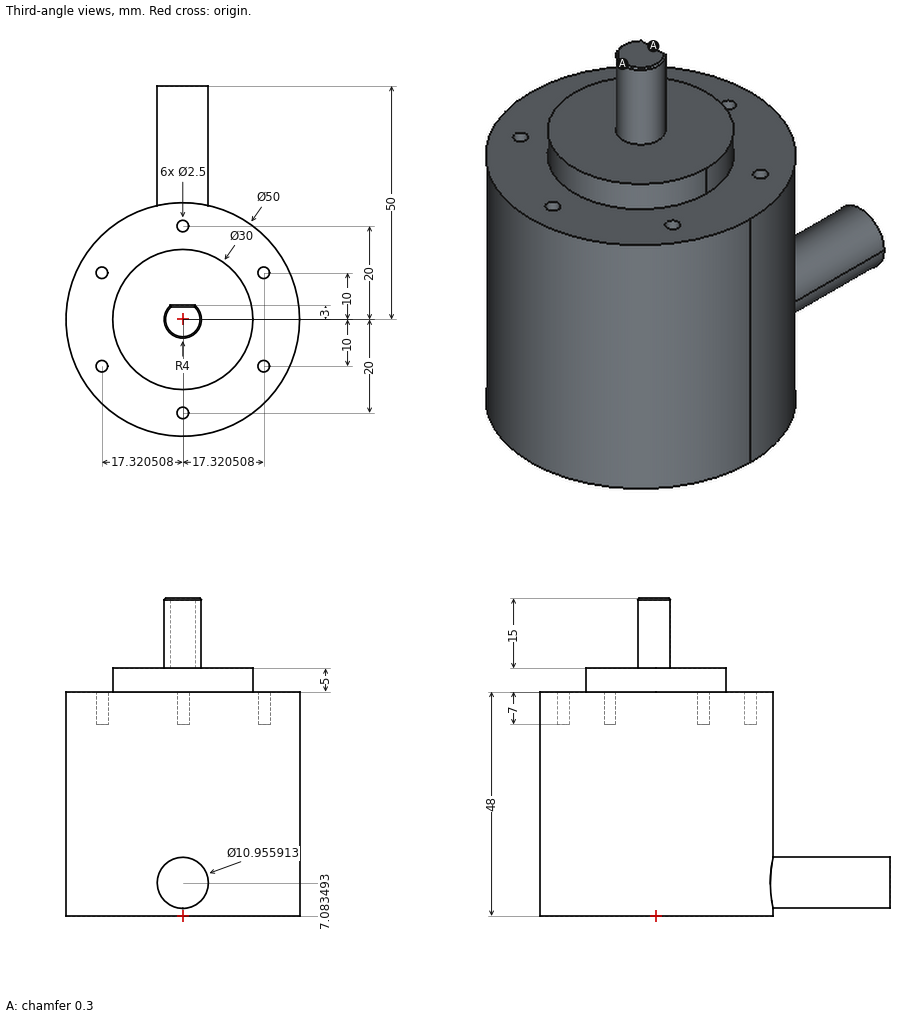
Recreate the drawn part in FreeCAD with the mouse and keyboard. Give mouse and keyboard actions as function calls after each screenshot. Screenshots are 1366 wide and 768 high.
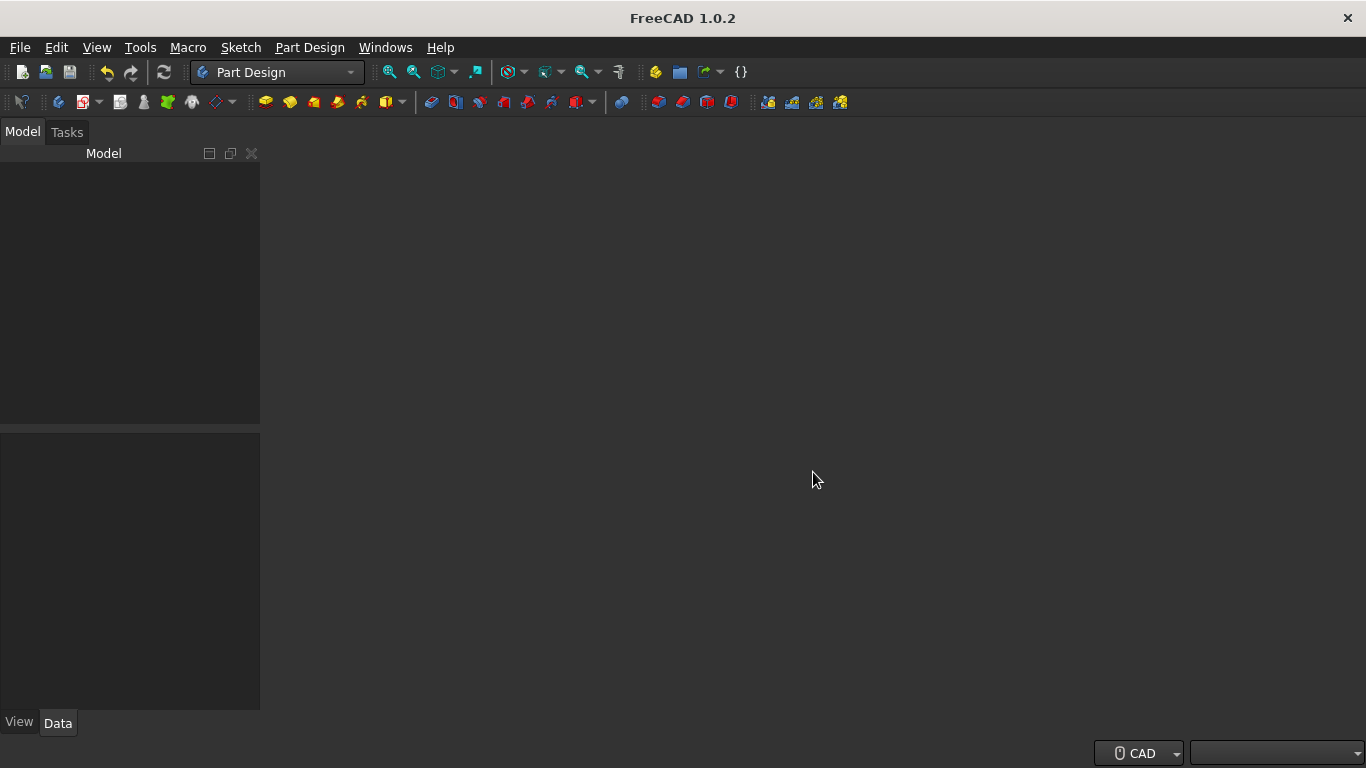
click(22, 72)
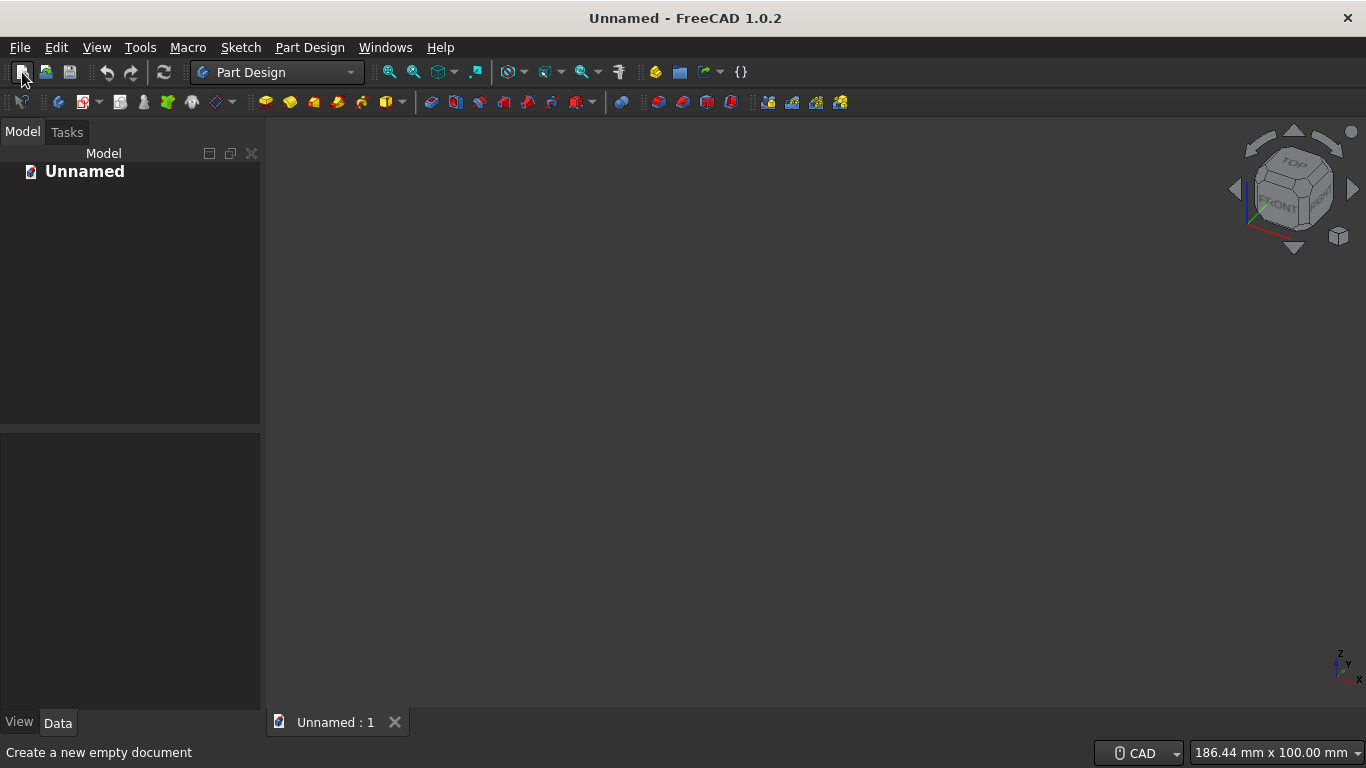
click(84, 102)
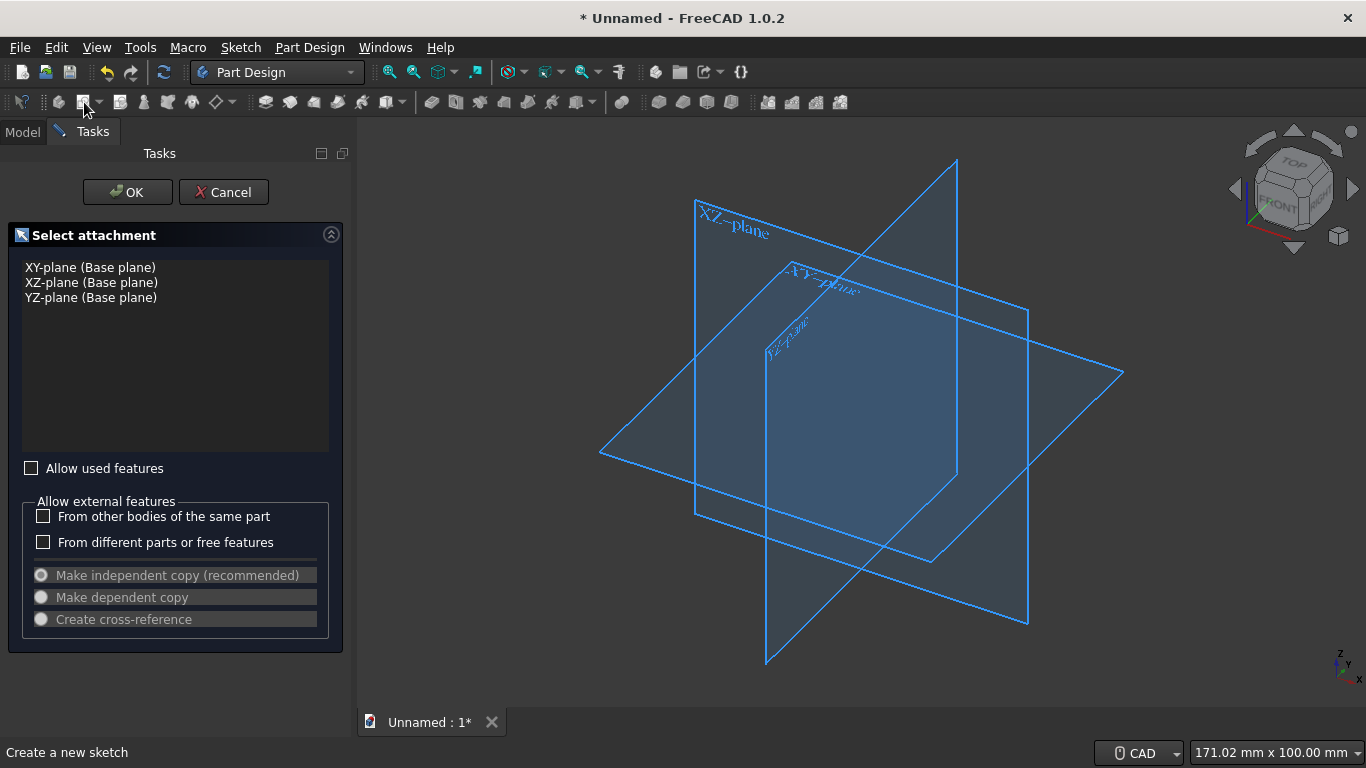
click(82, 268)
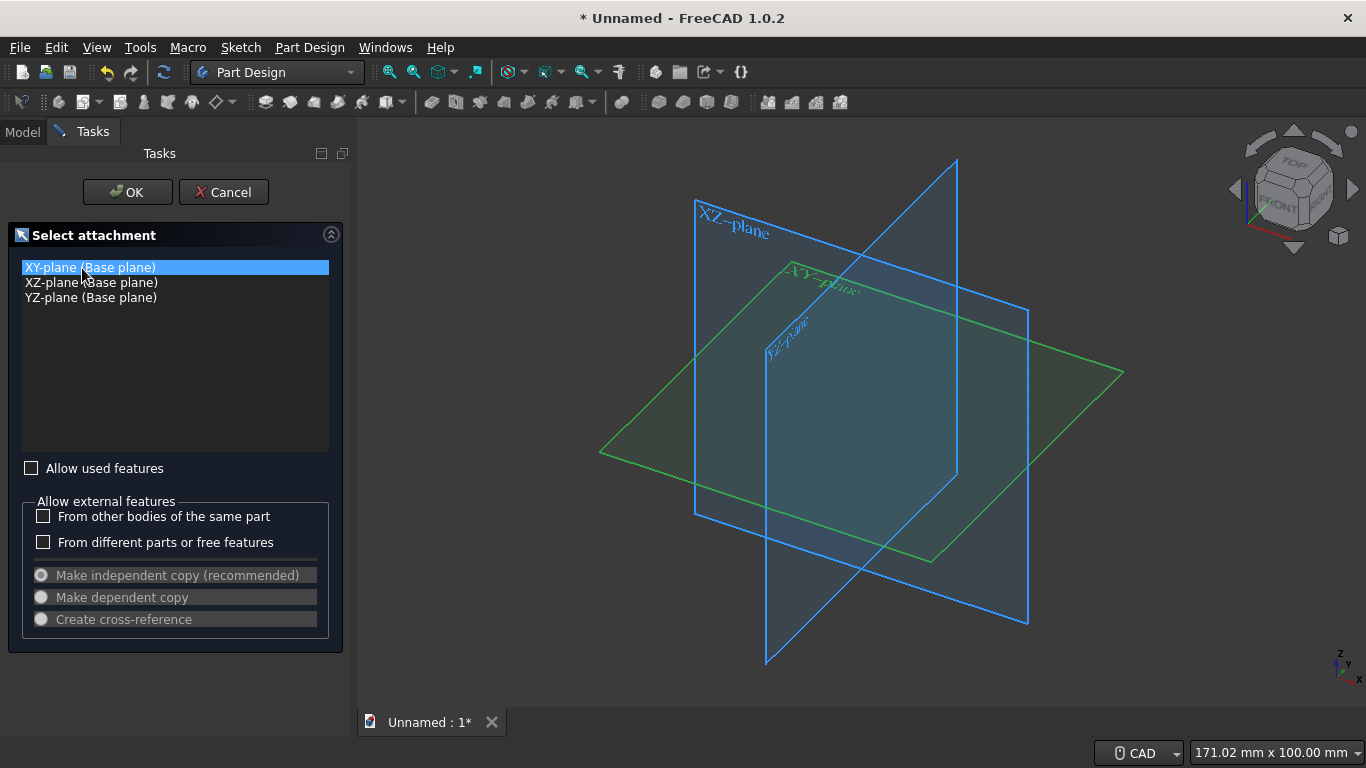
click(128, 192)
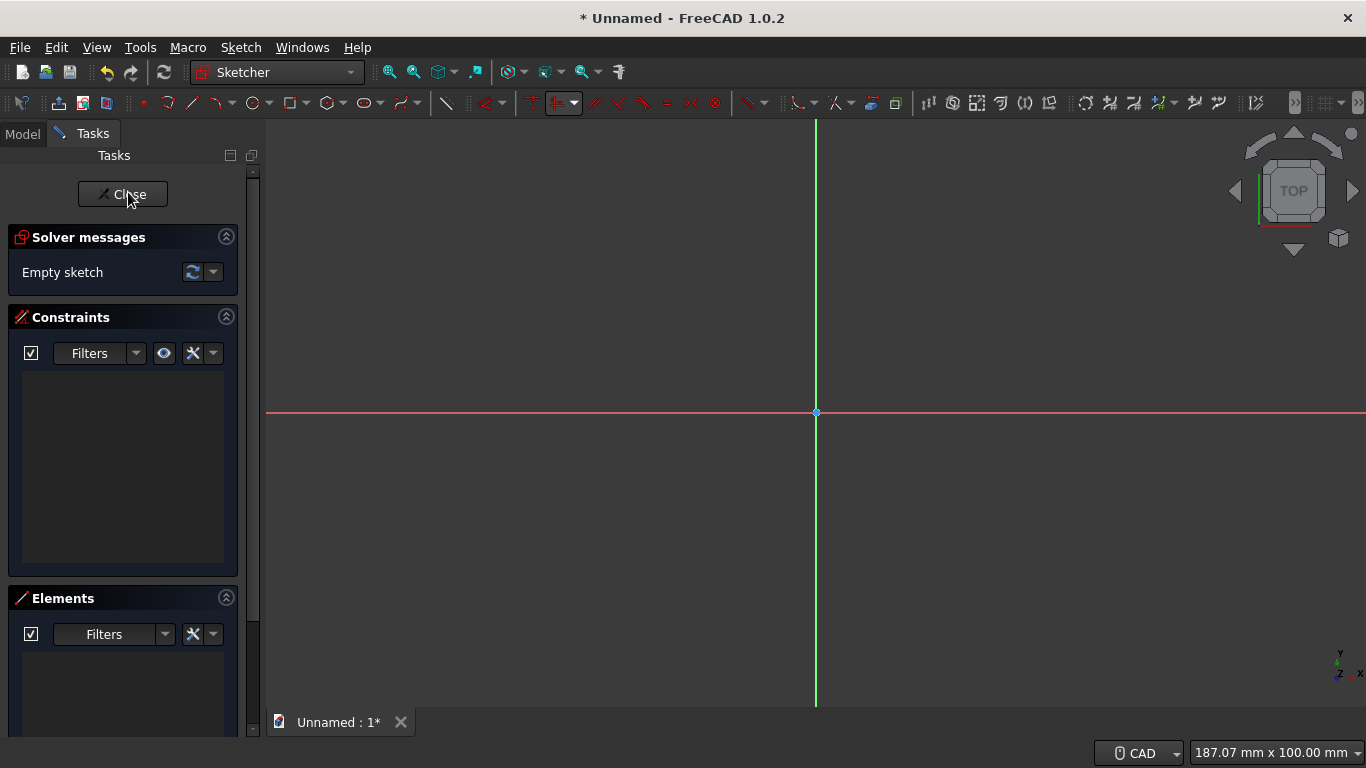
click(254, 104)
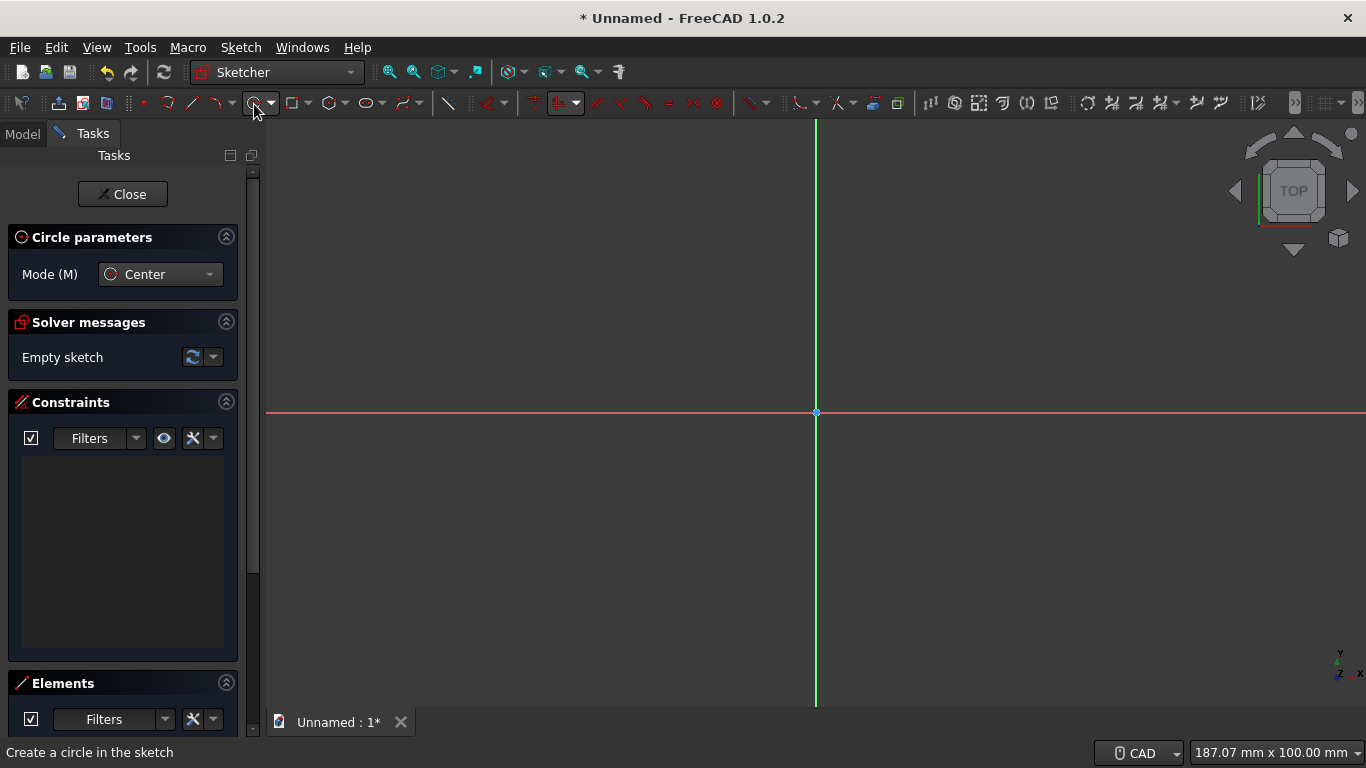
click(816, 413)
move(920, 309)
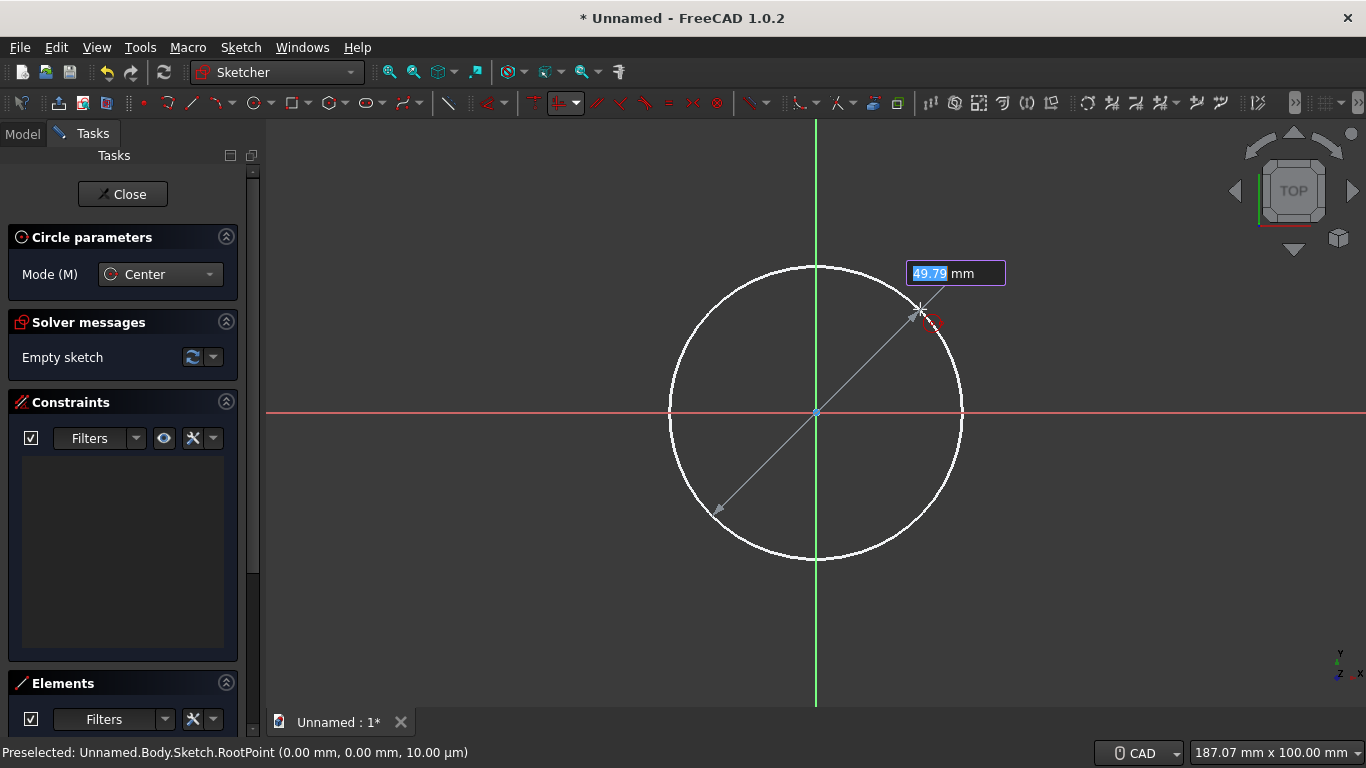
text(50)
key(Return)
key(Escape)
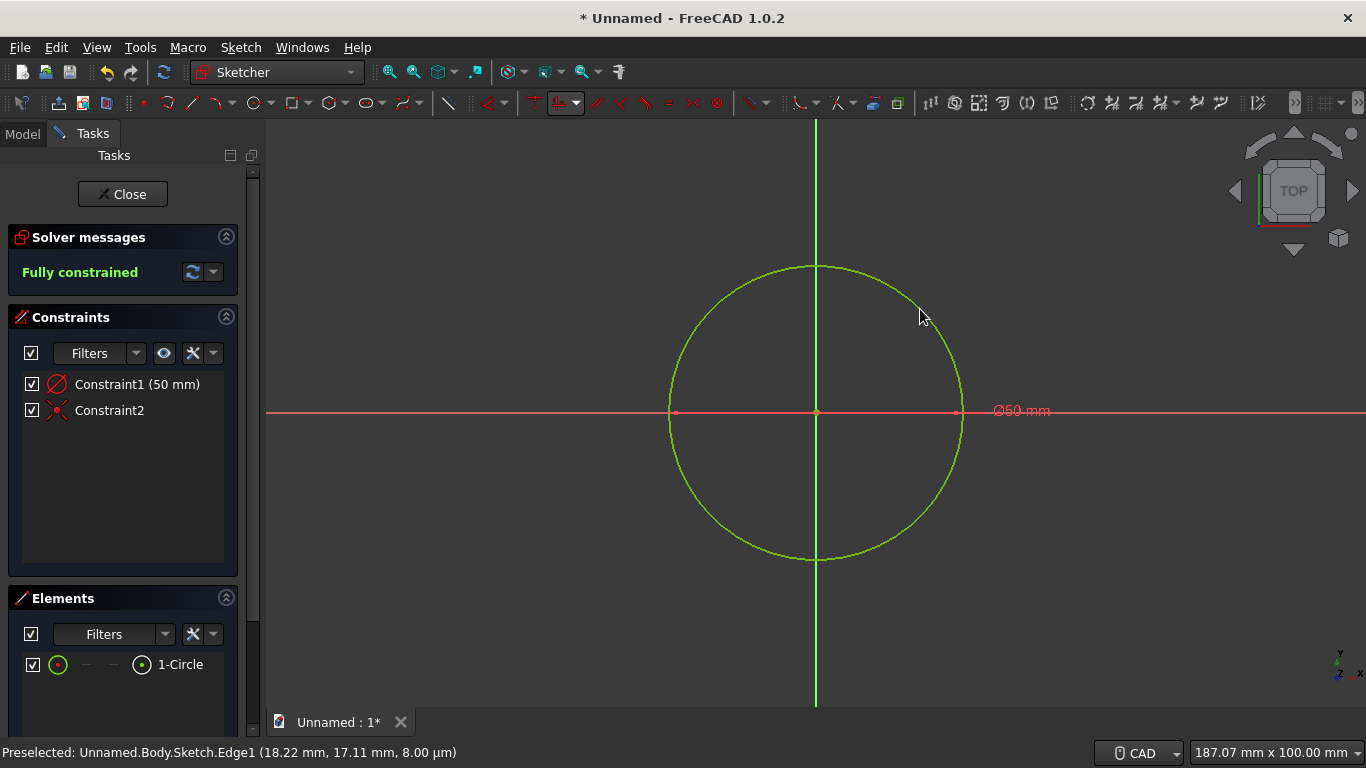
click(123, 194)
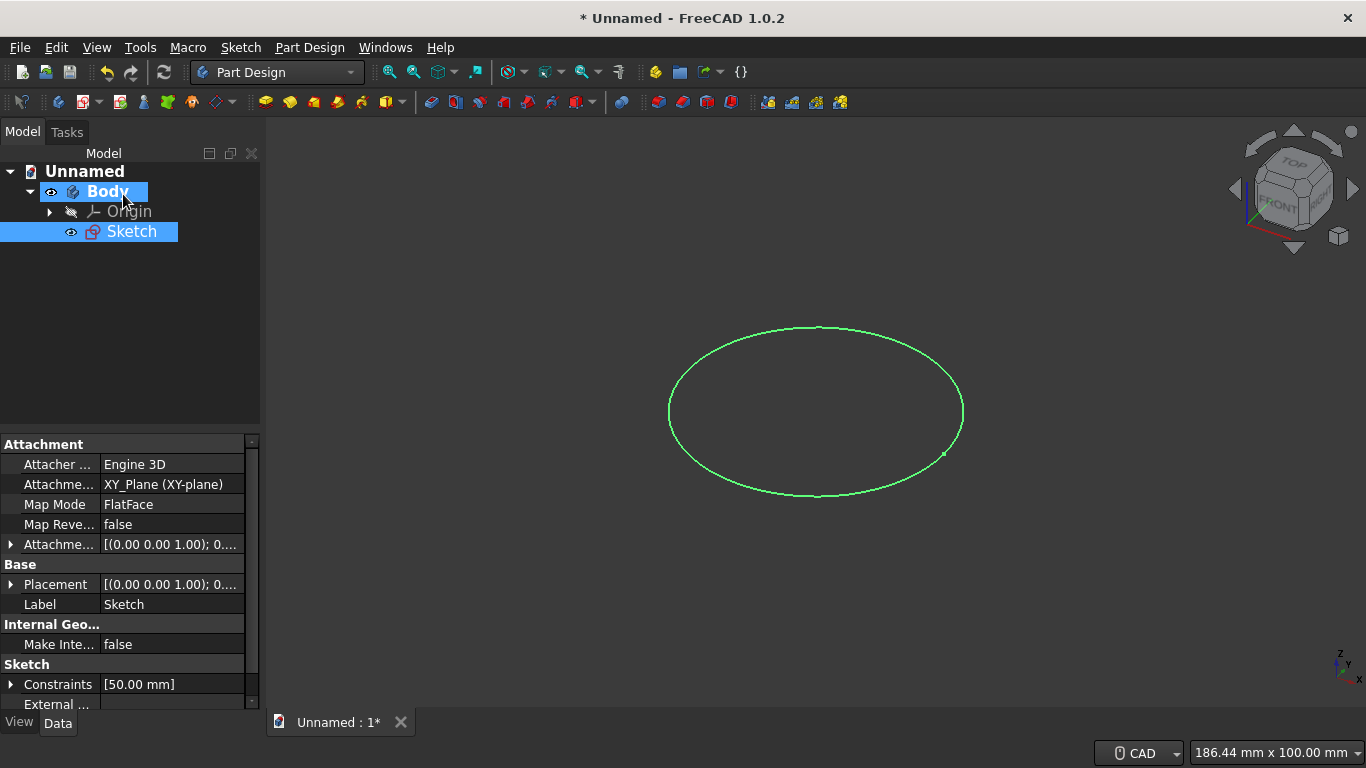
click(266, 102)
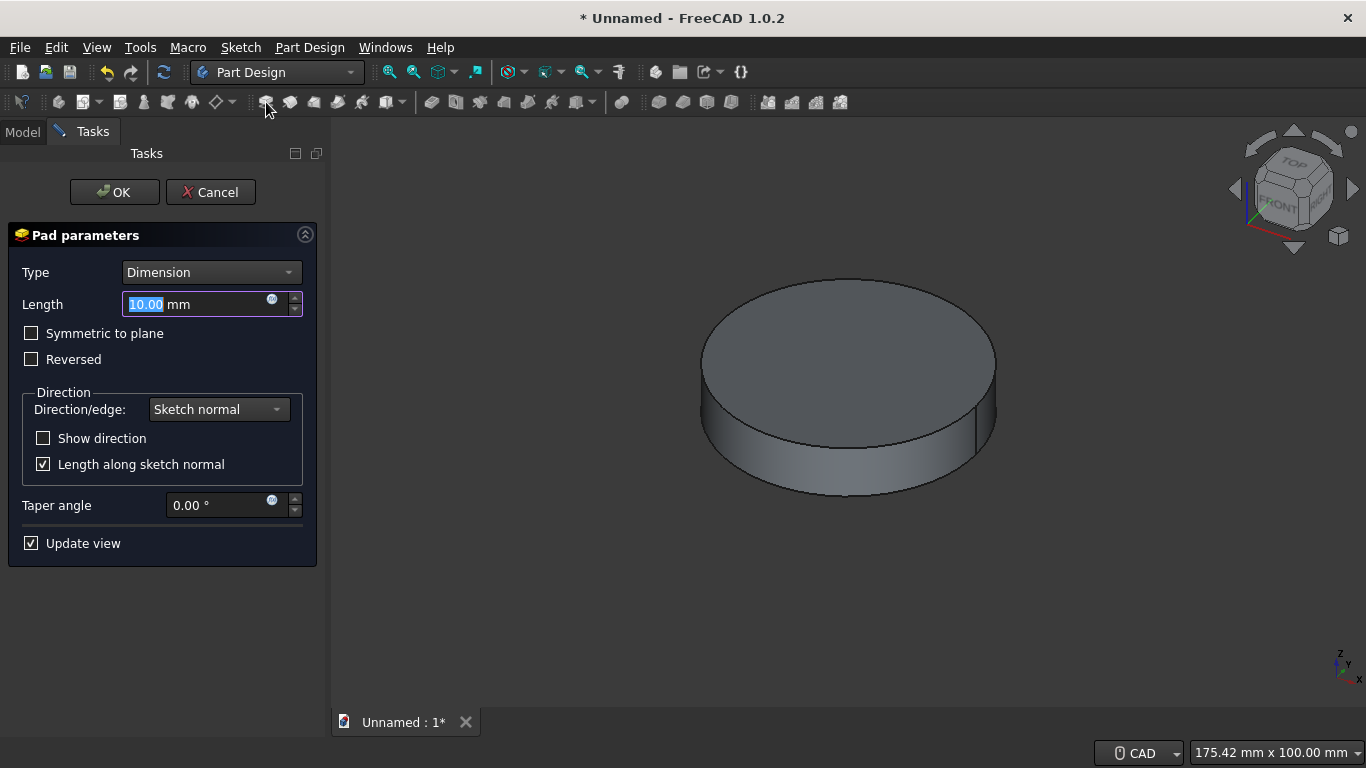
text(48)
key(Tab)